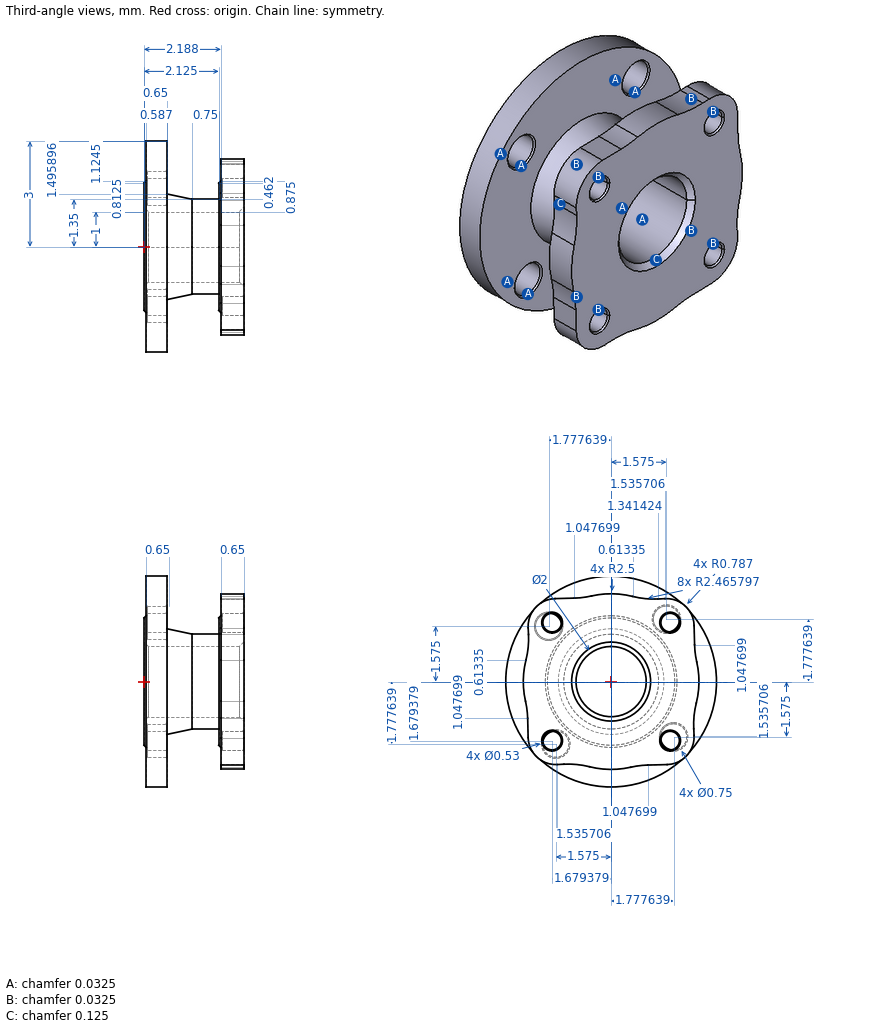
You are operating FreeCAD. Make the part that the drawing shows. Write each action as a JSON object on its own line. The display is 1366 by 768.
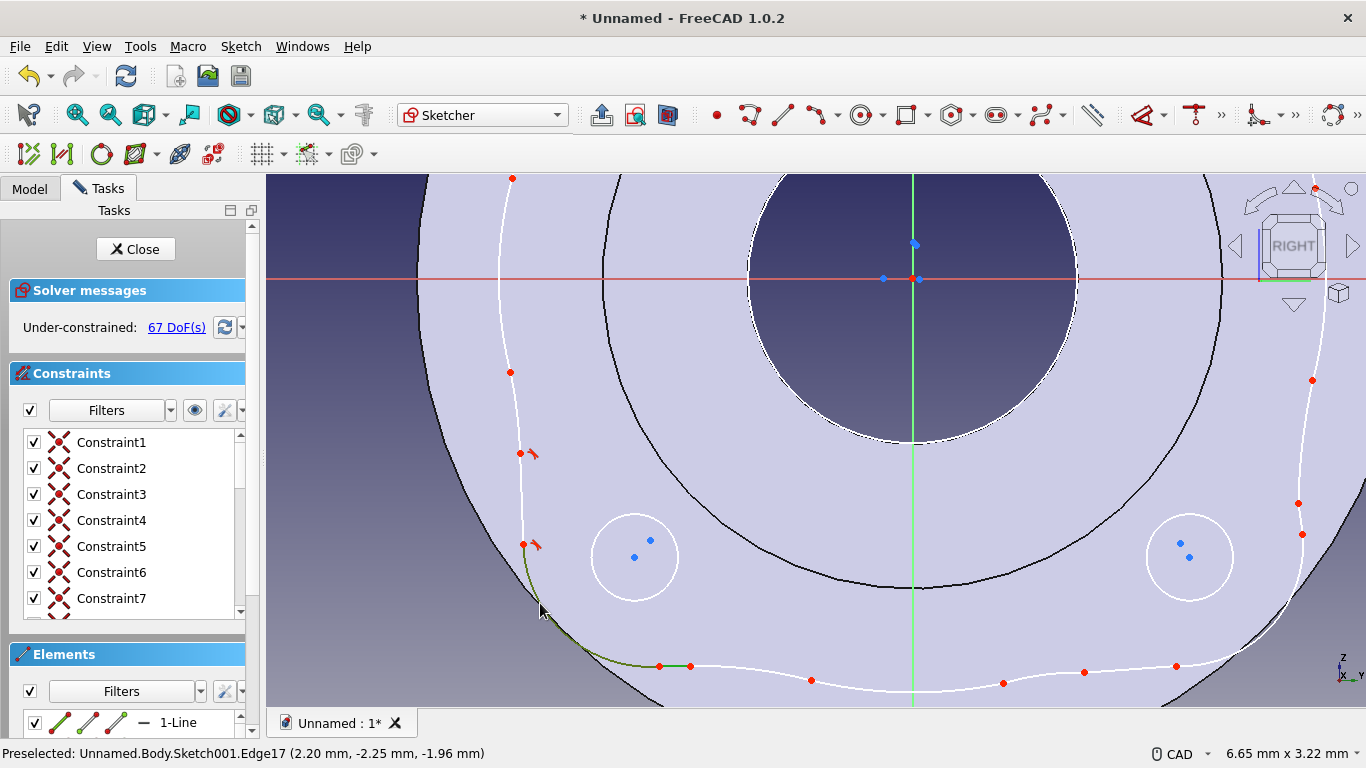
{"action": "key", "text": "t"}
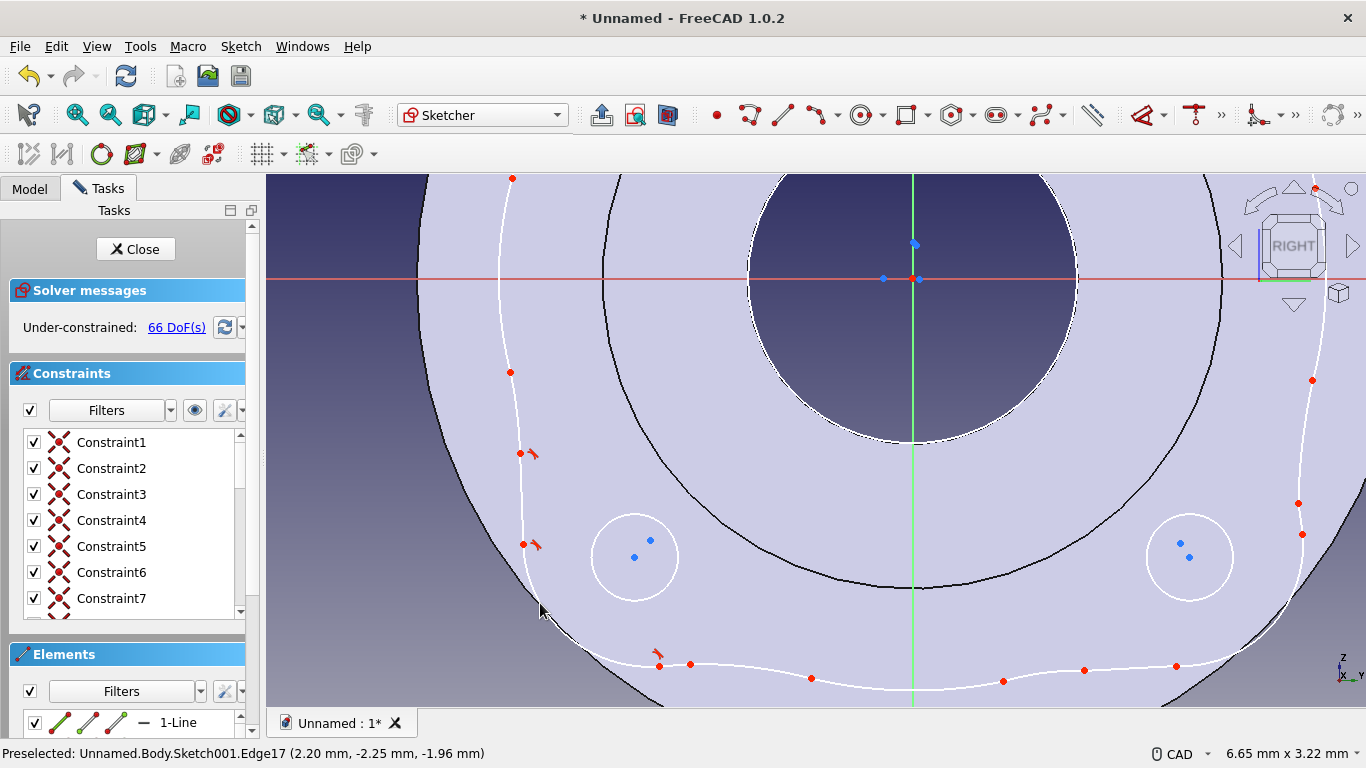
{"action": "scroll", "coordinate": [669, 666], "scroll_direction": "up", "scroll_amount": 2}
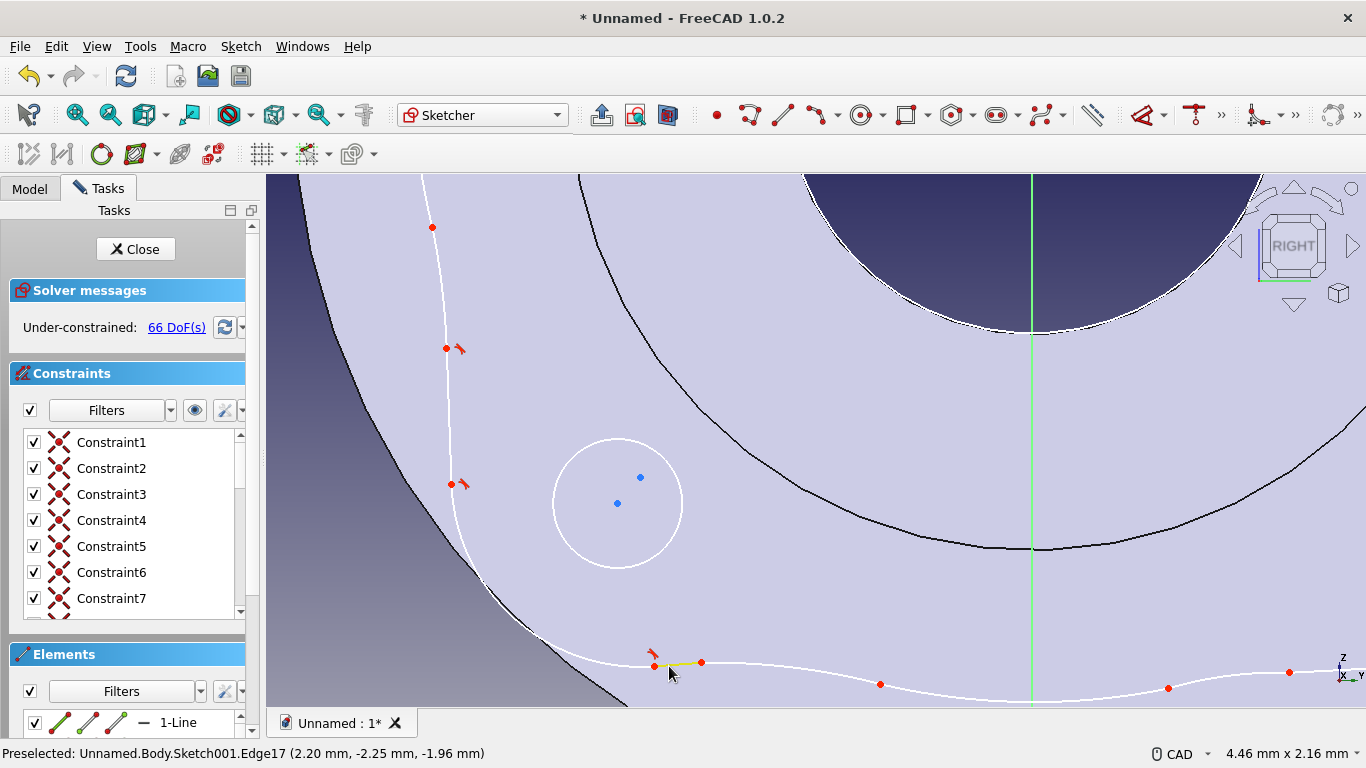
{"action": "left_click", "coordinate": [669, 665]}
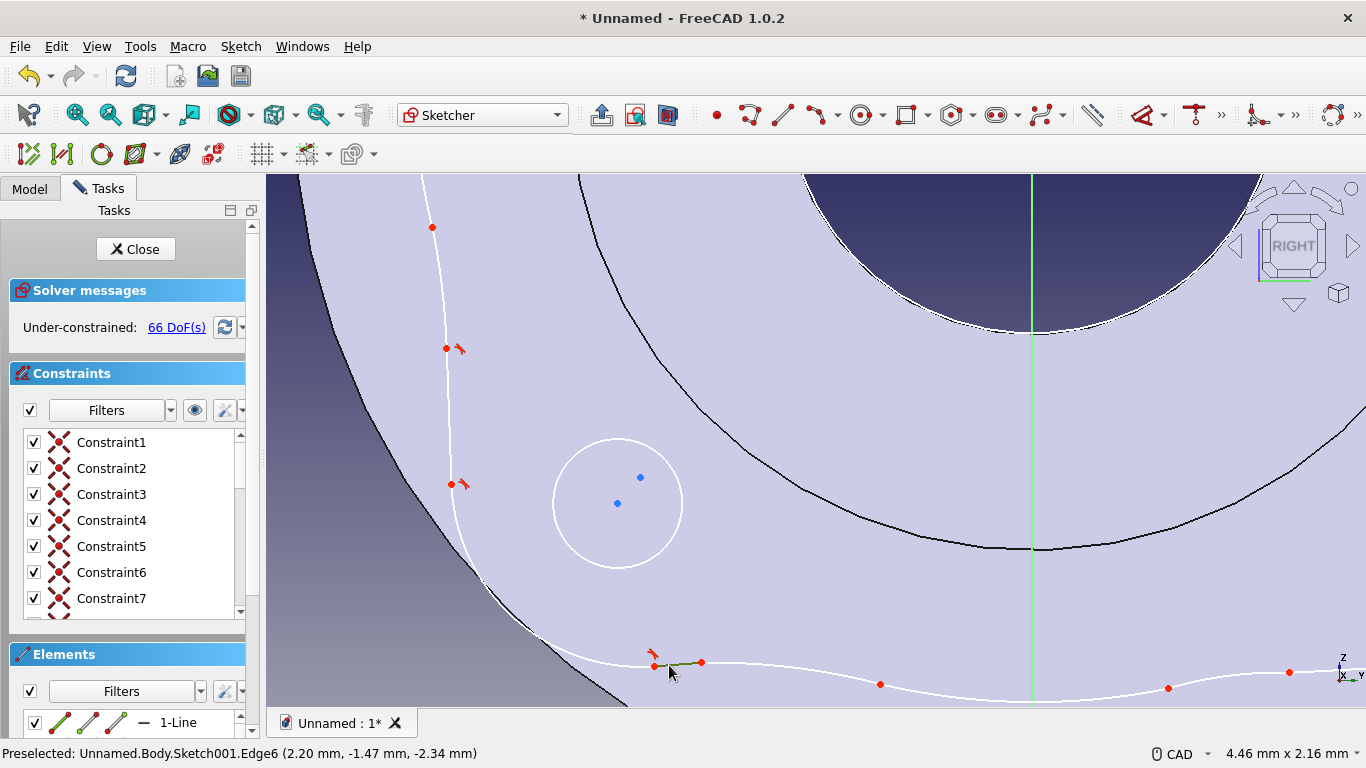
{"action": "scroll", "coordinate": [625, 593], "scroll_direction": "down", "scroll_amount": 6}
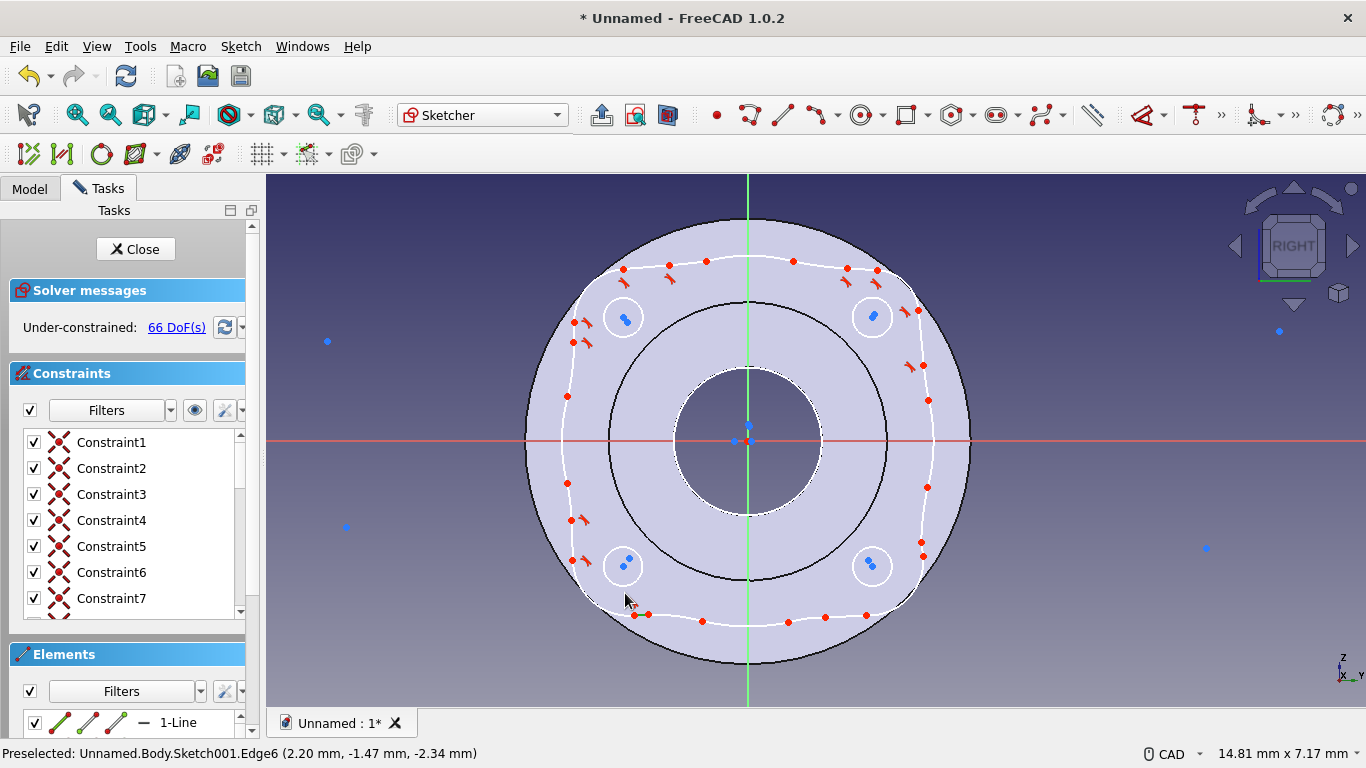
{"action": "left_click", "coordinate": [686, 618]}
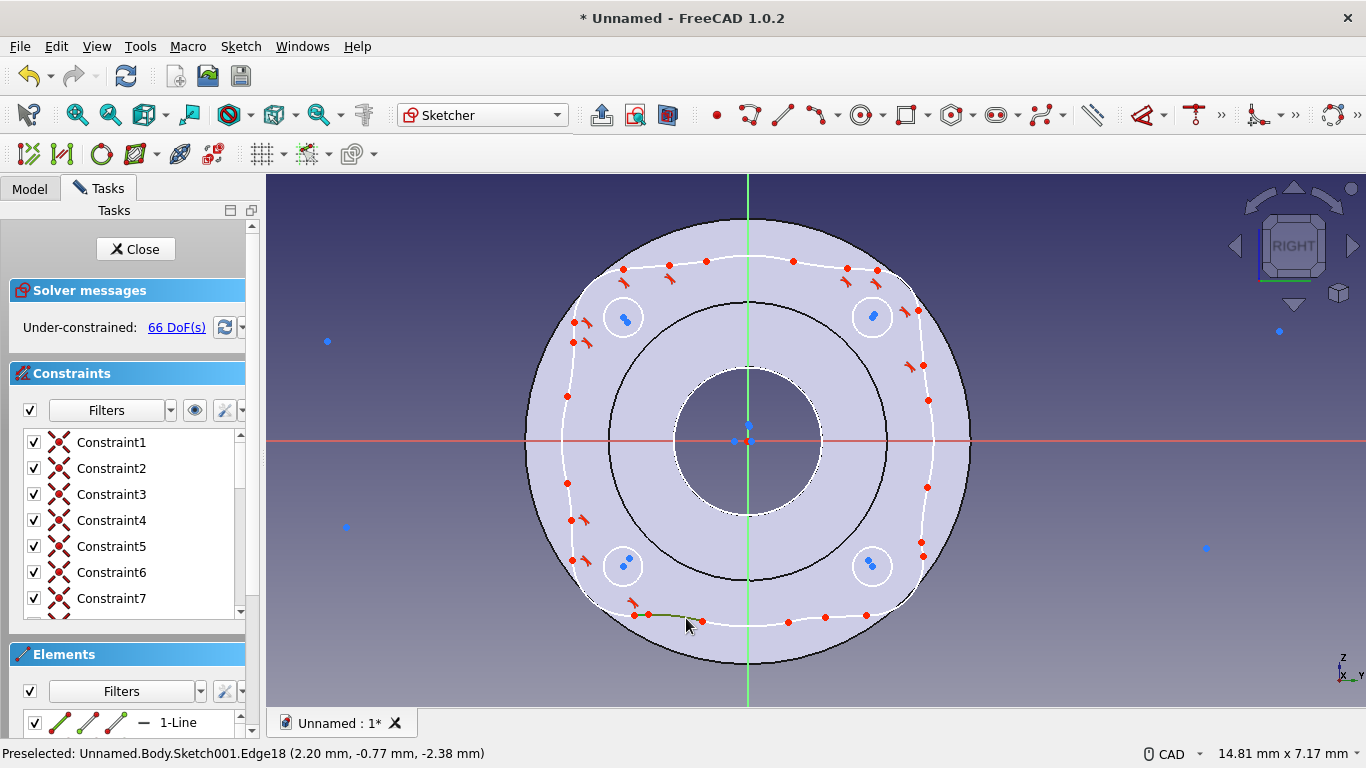
{"action": "key", "text": "t"}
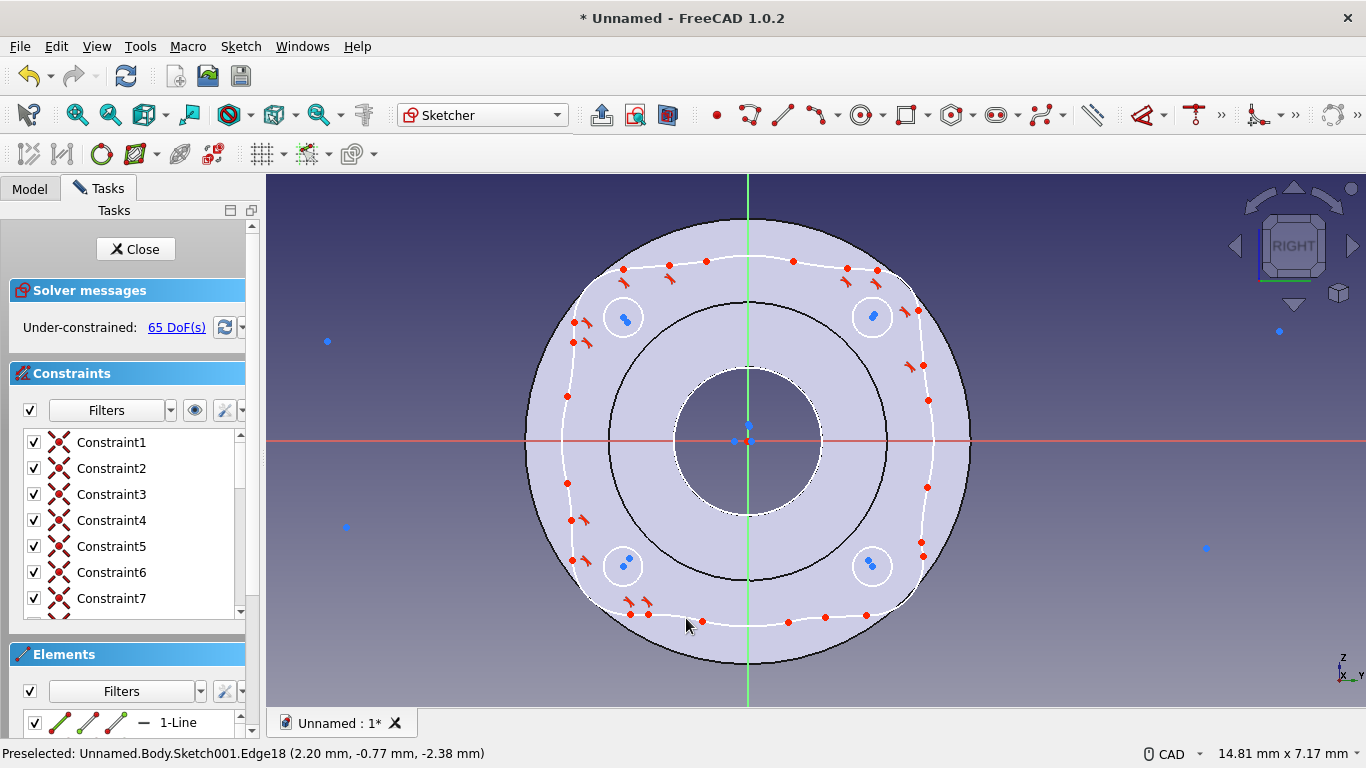
{"action": "left_click", "coordinate": [838, 617]}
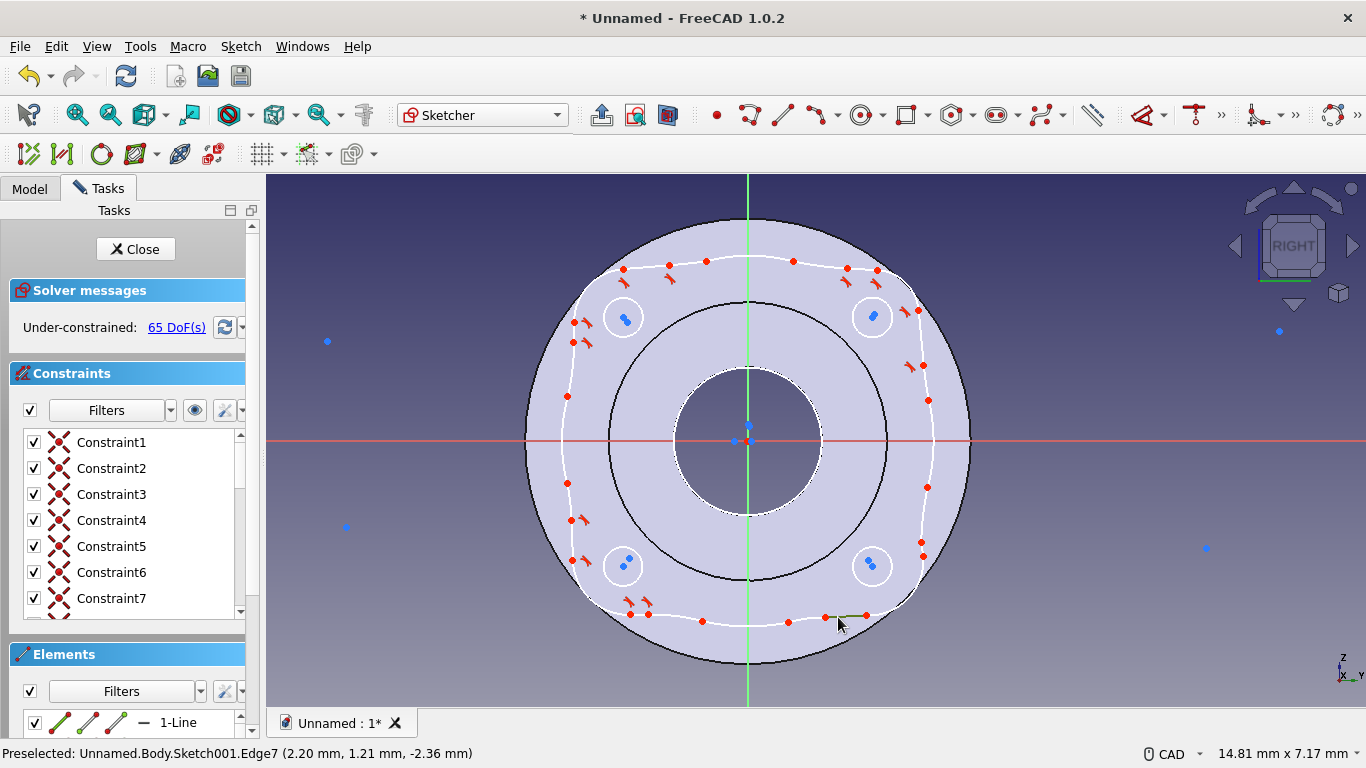
{"action": "scroll", "coordinate": [814, 618], "scroll_direction": "up", "scroll_amount": 2}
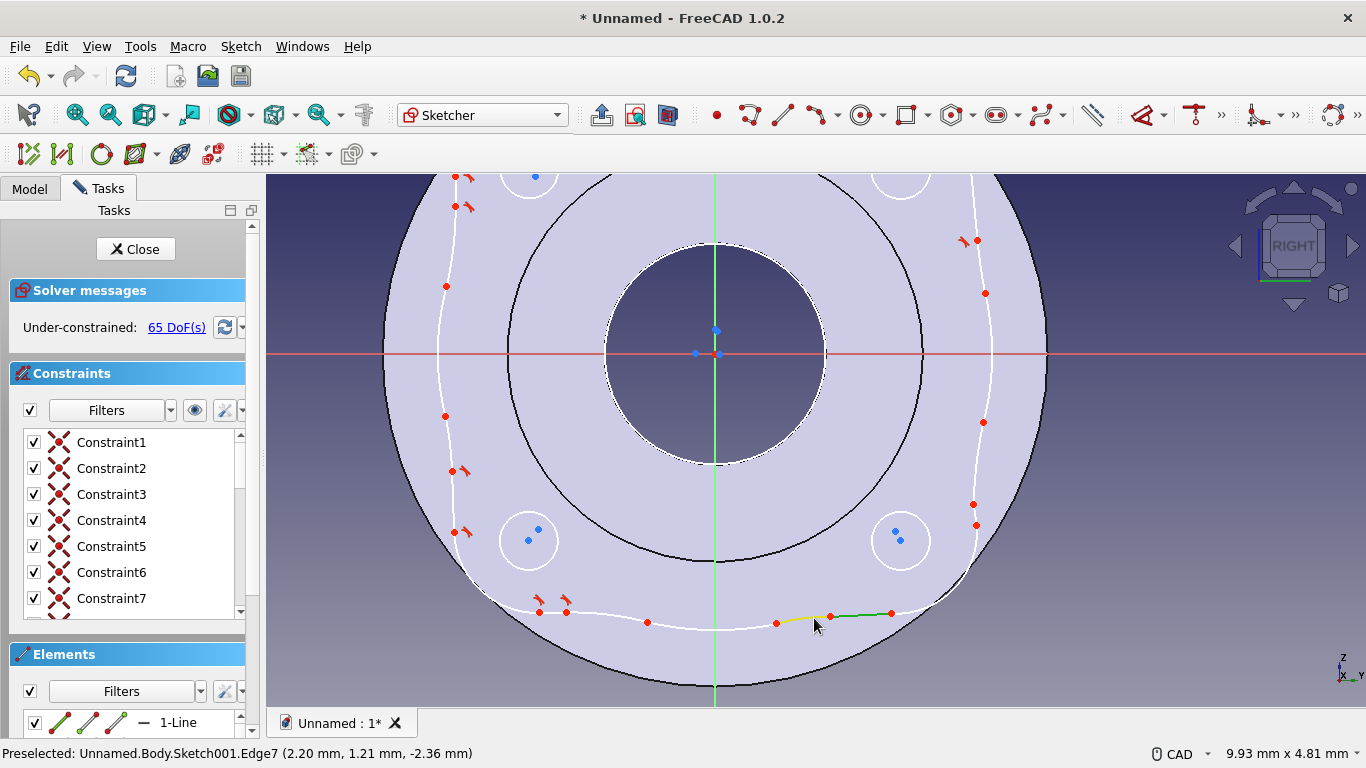
{"action": "left_click", "coordinate": [814, 617]}